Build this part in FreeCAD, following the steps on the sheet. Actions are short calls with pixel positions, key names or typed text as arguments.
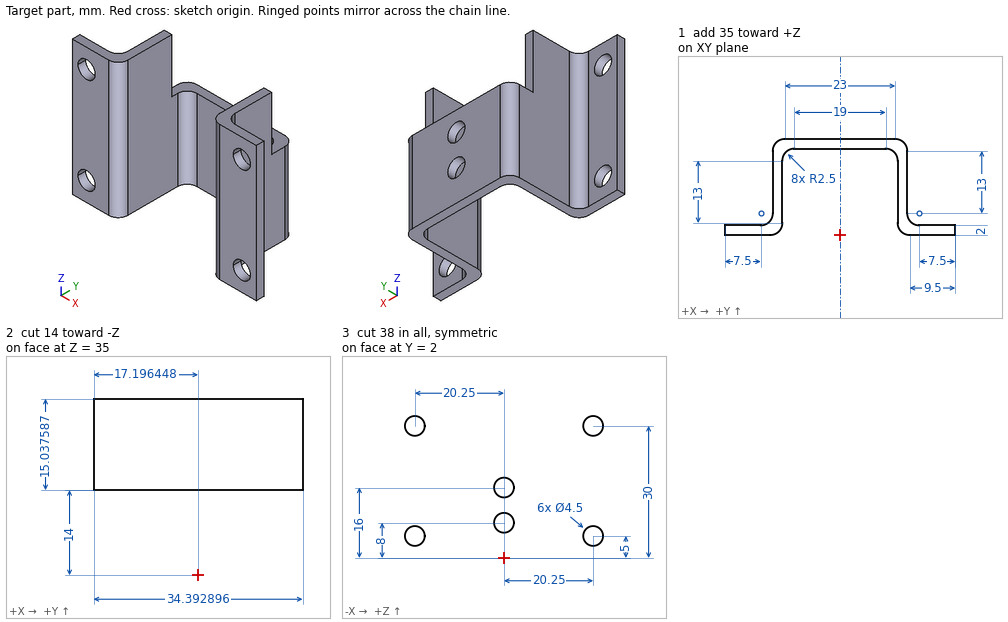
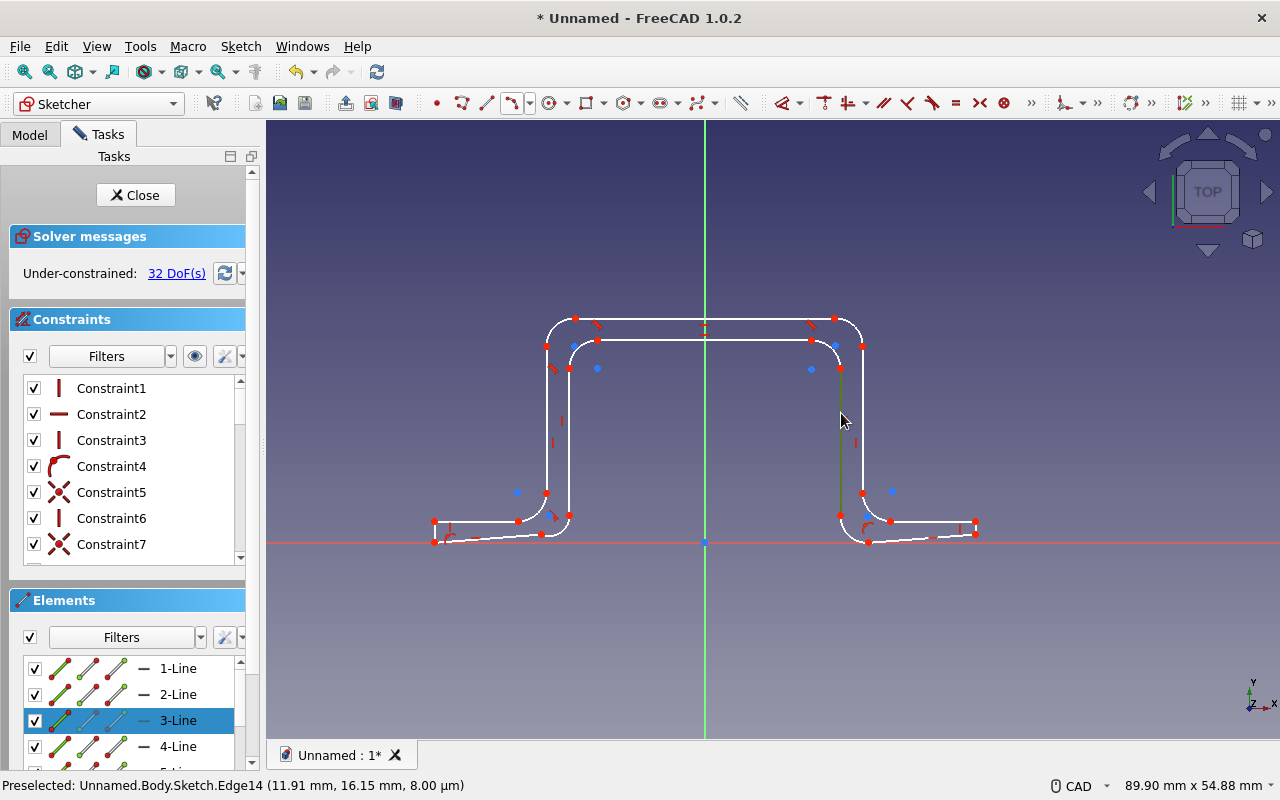
click(837, 356)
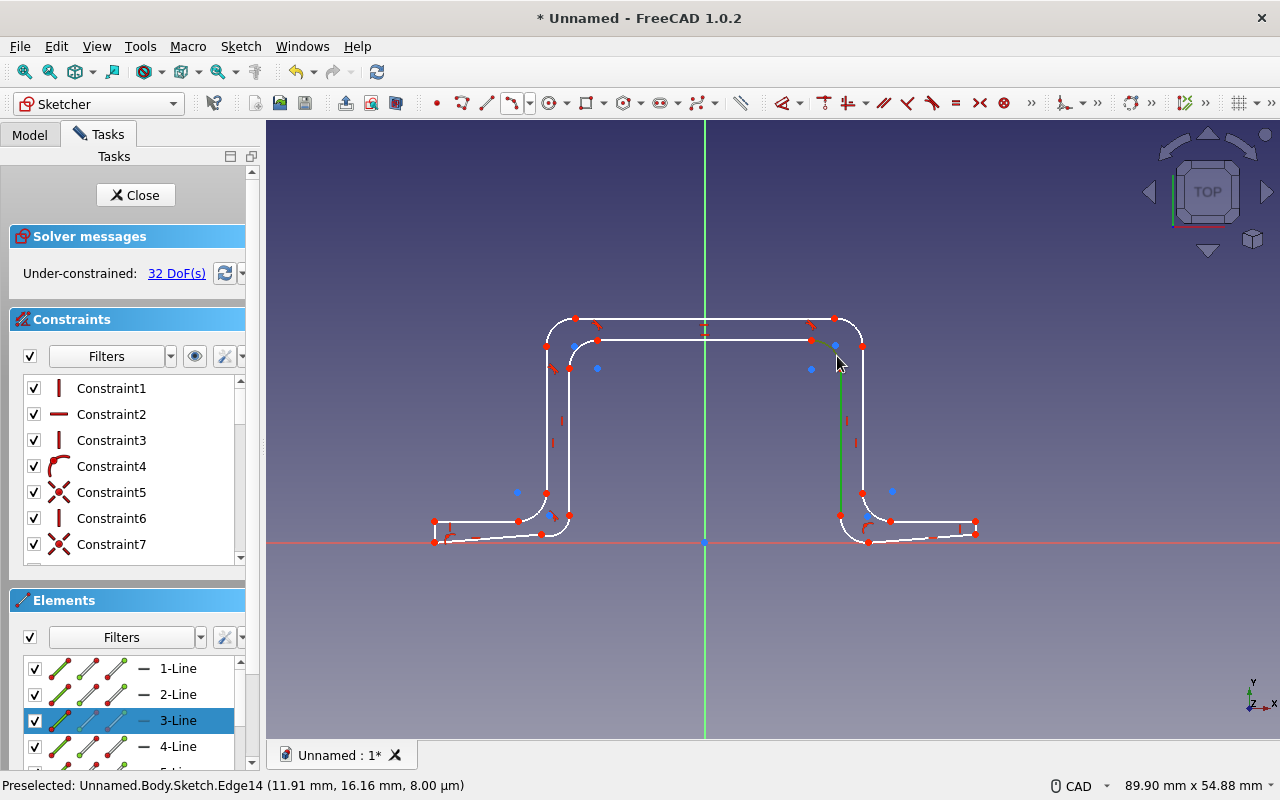
click(932, 104)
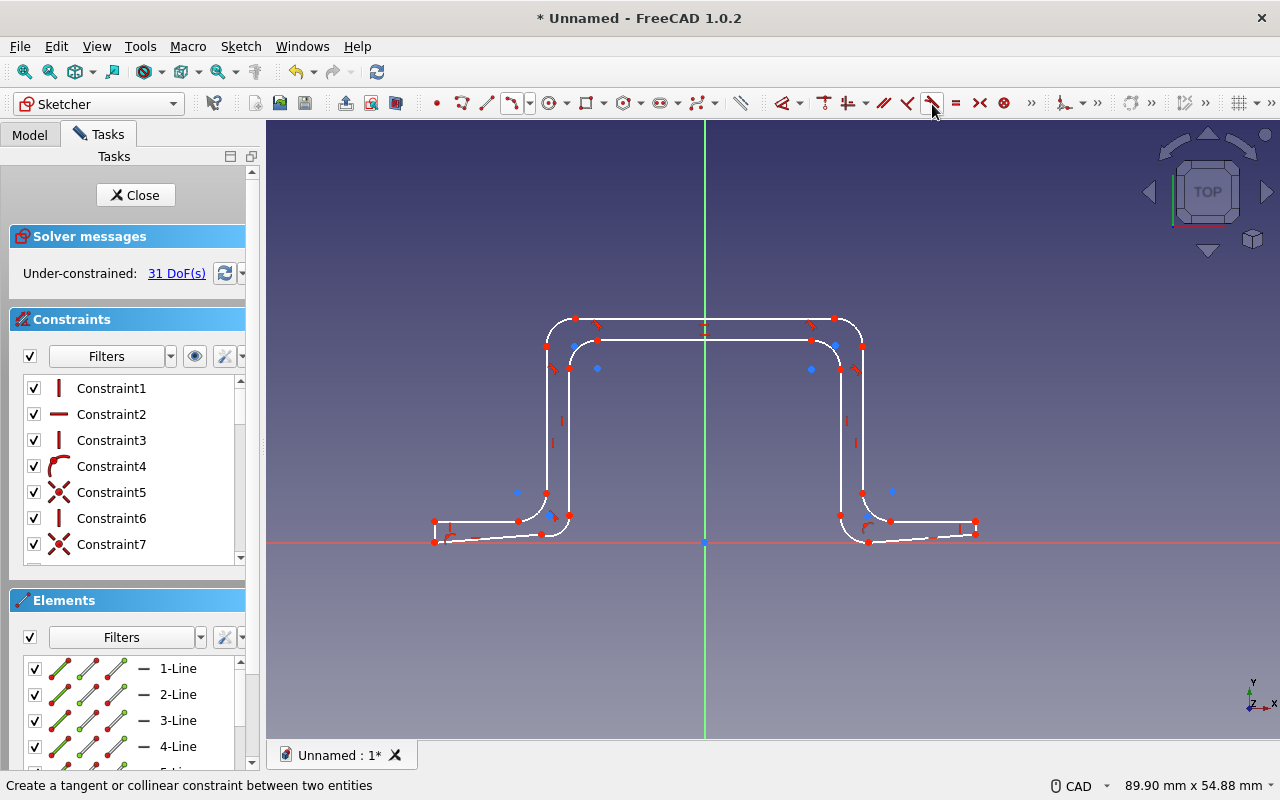
click(841, 413)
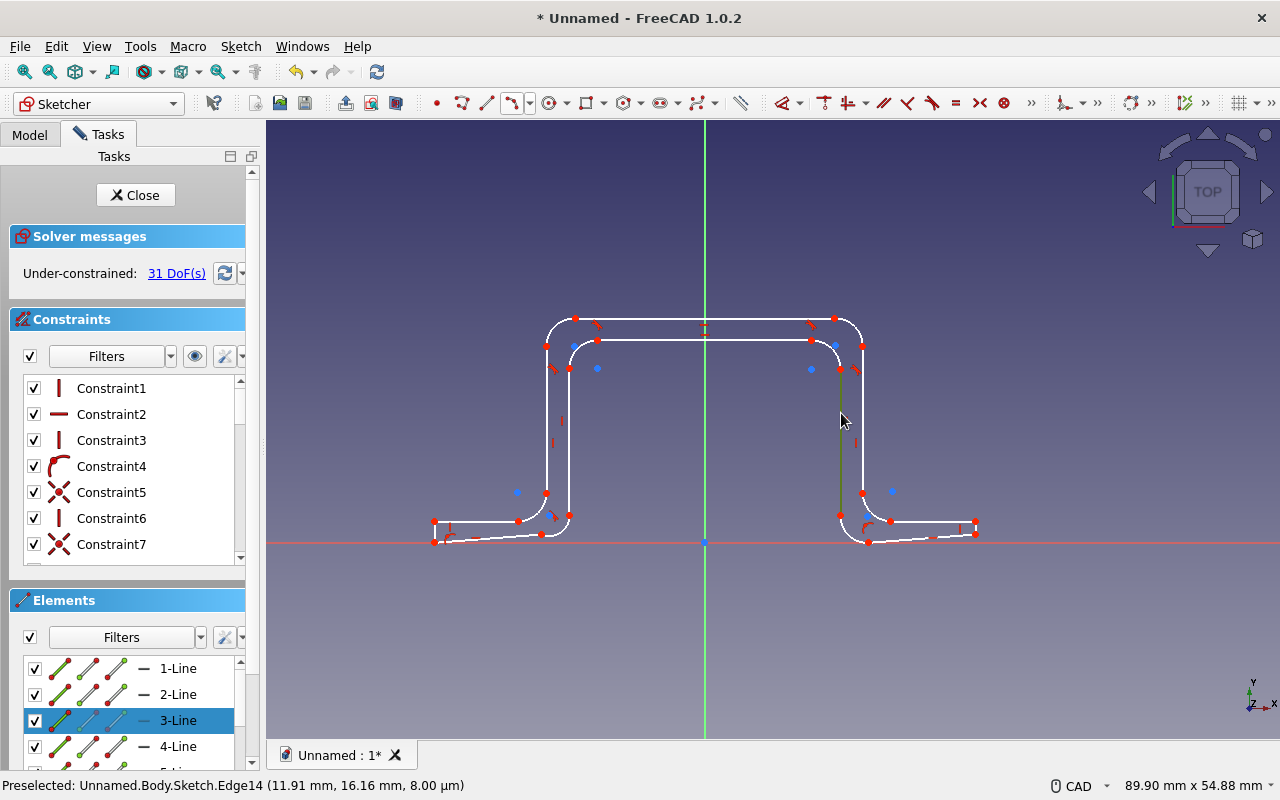
click(843, 528)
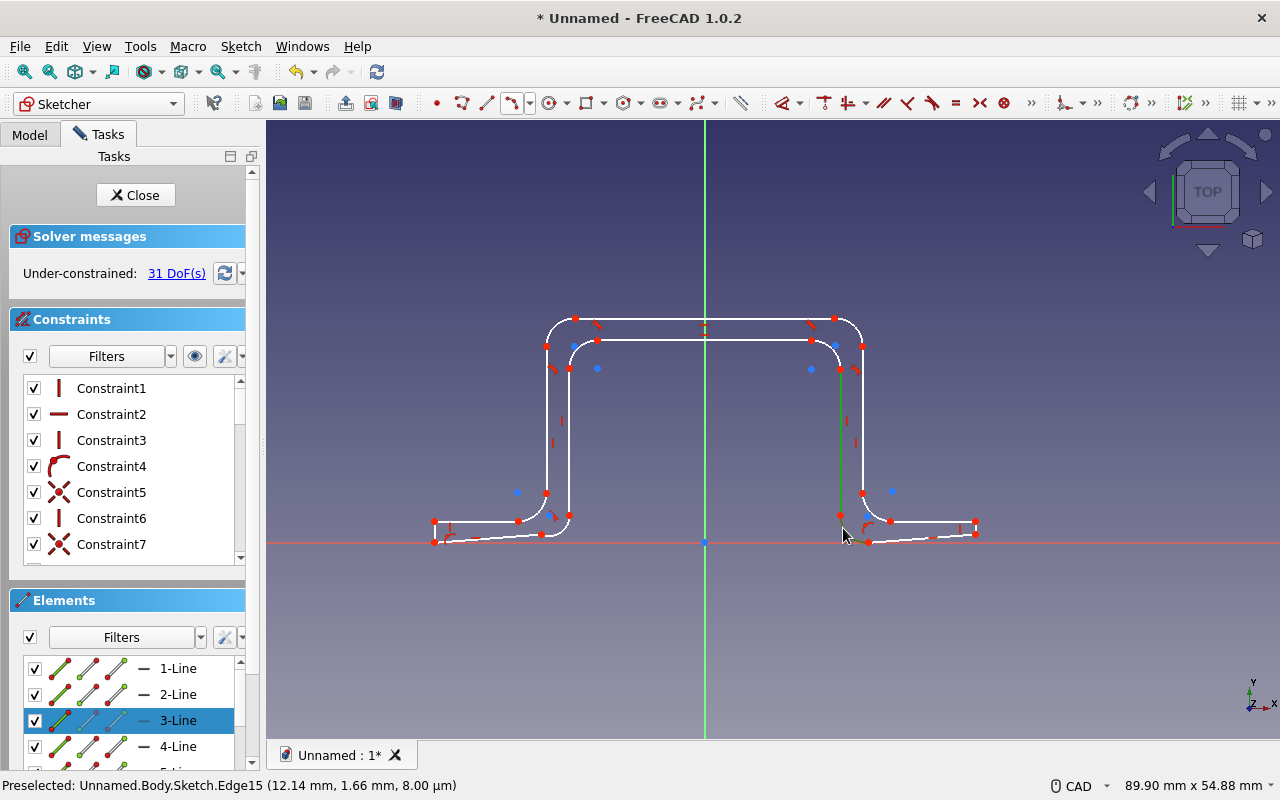
click(932, 104)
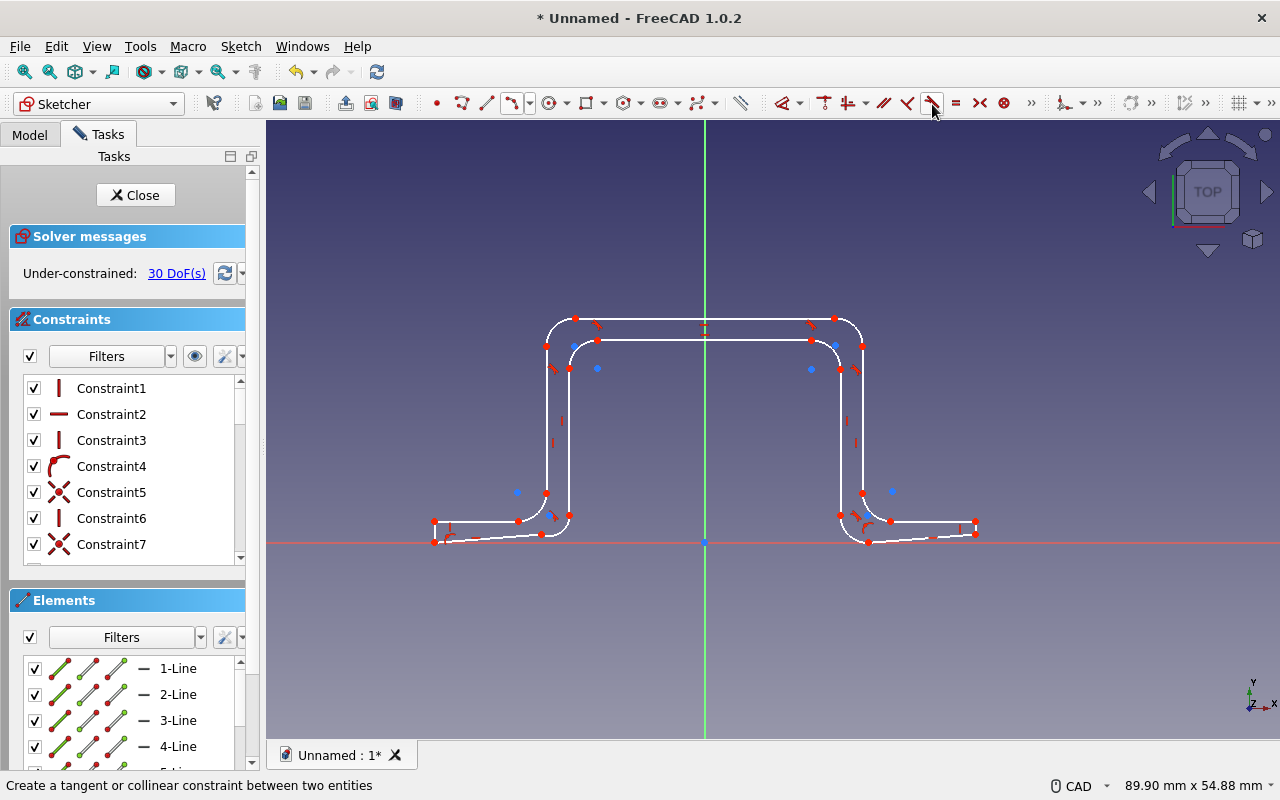
click(901, 540)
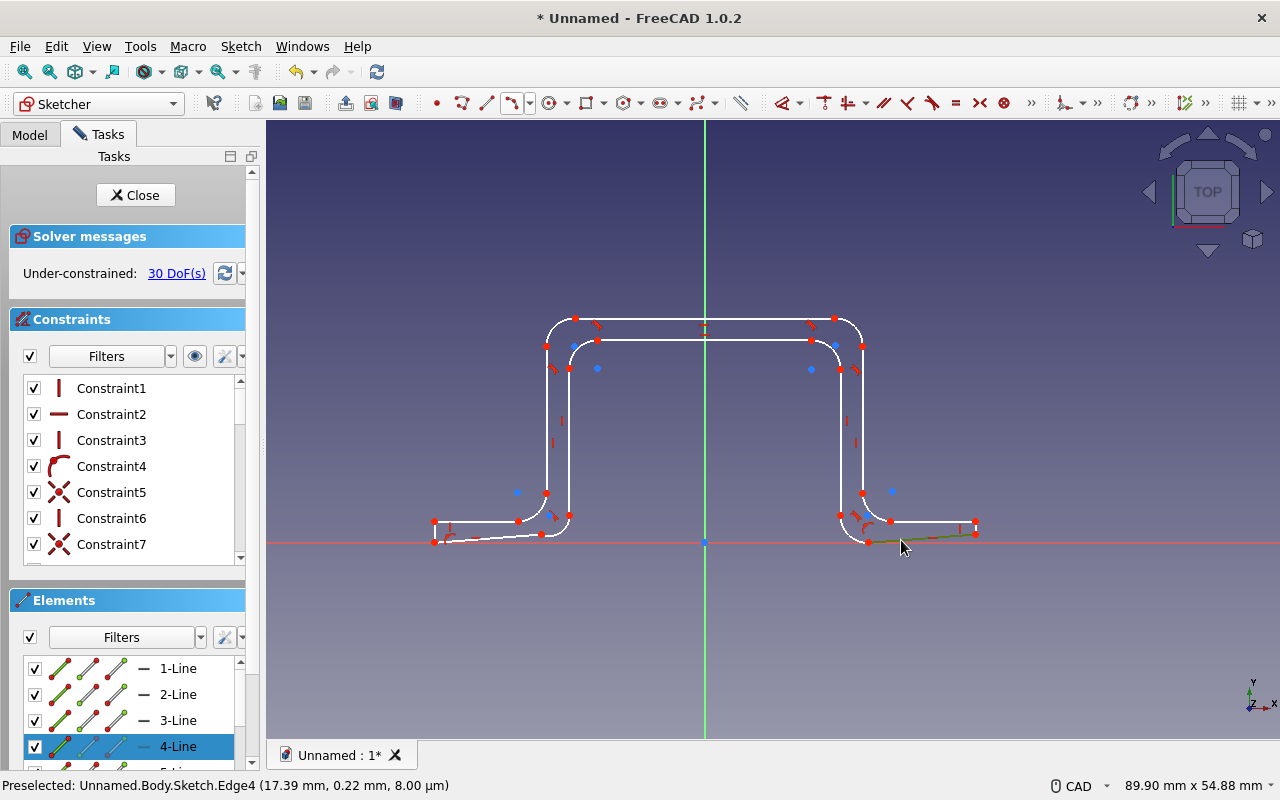
click(844, 528)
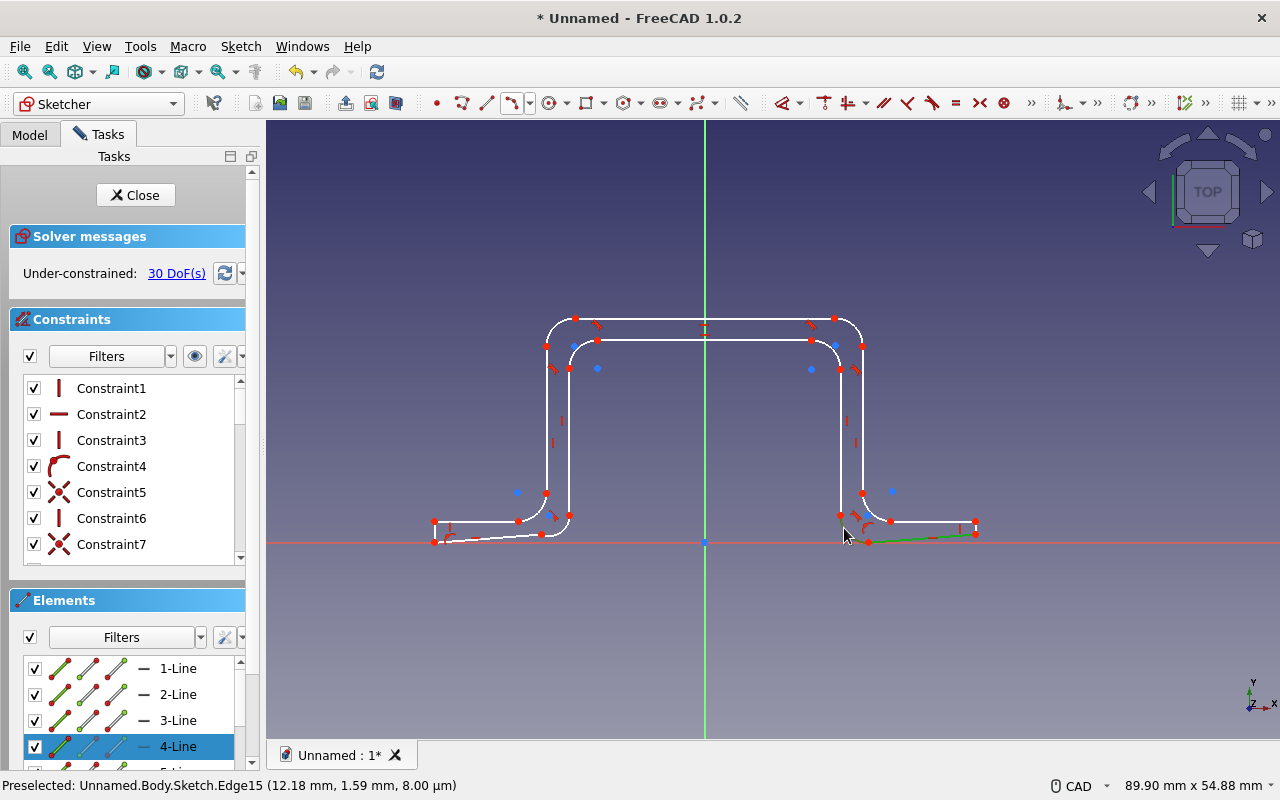
click(932, 104)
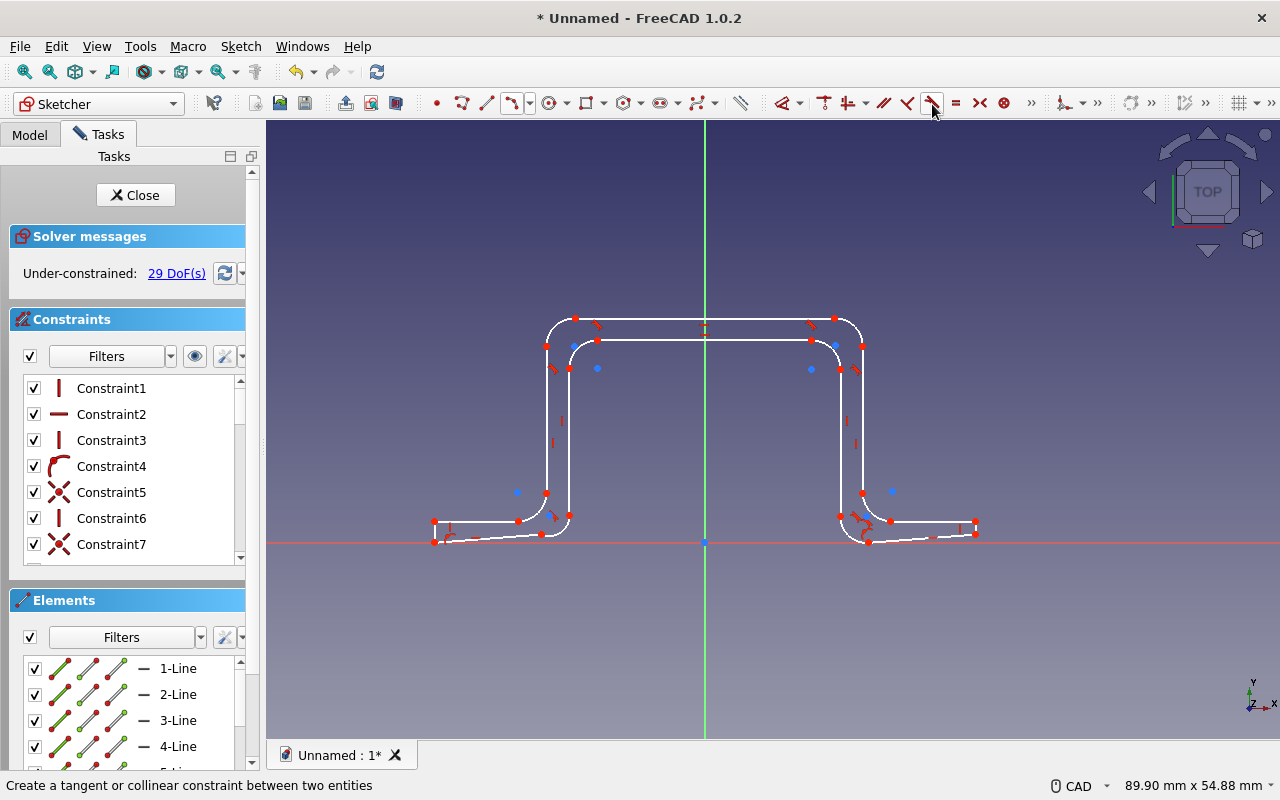
click(950, 522)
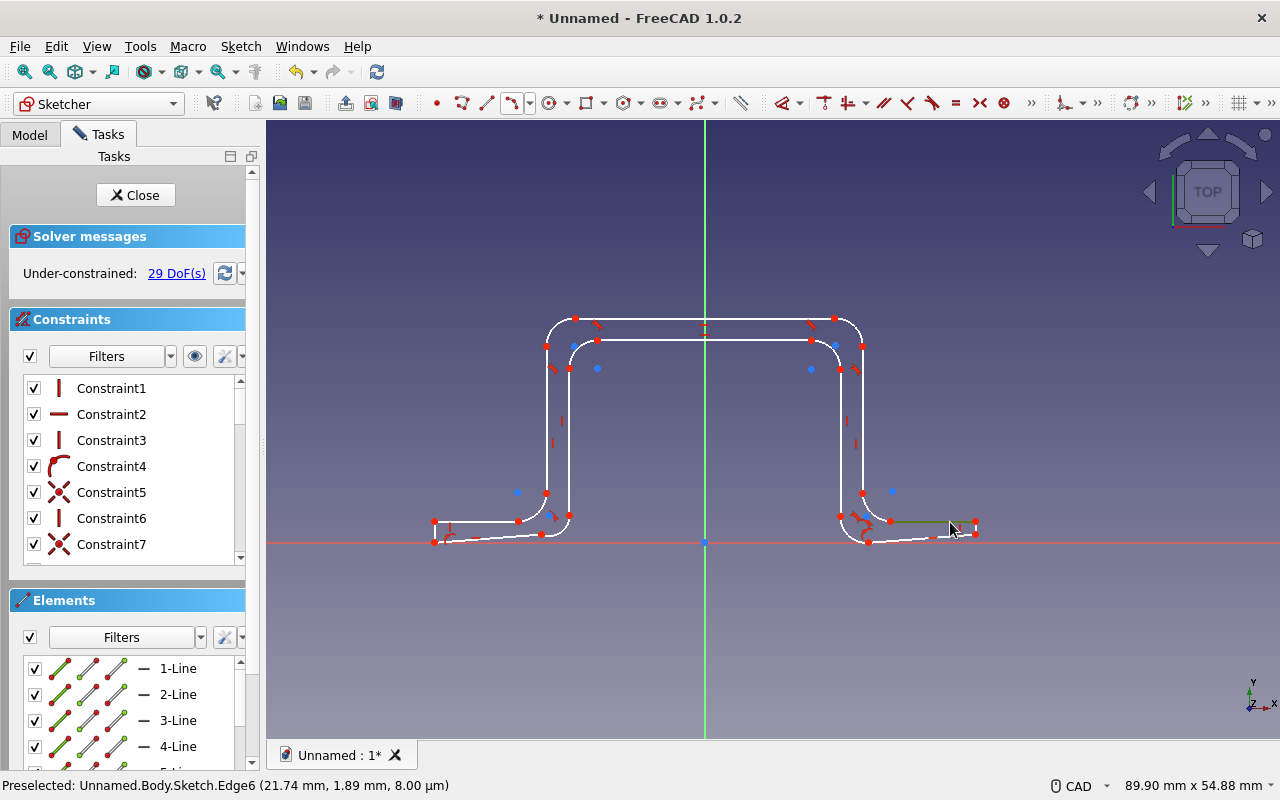
click(866, 506)